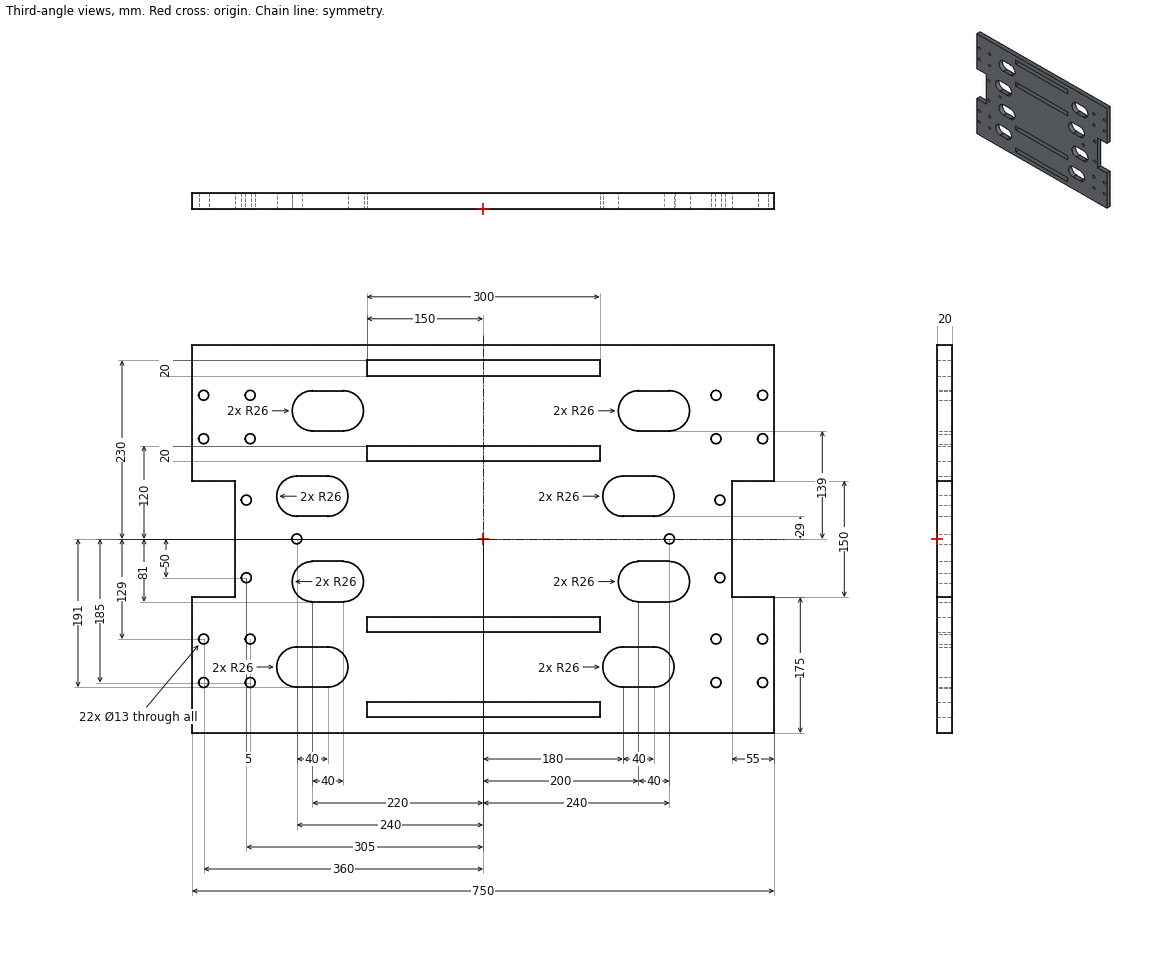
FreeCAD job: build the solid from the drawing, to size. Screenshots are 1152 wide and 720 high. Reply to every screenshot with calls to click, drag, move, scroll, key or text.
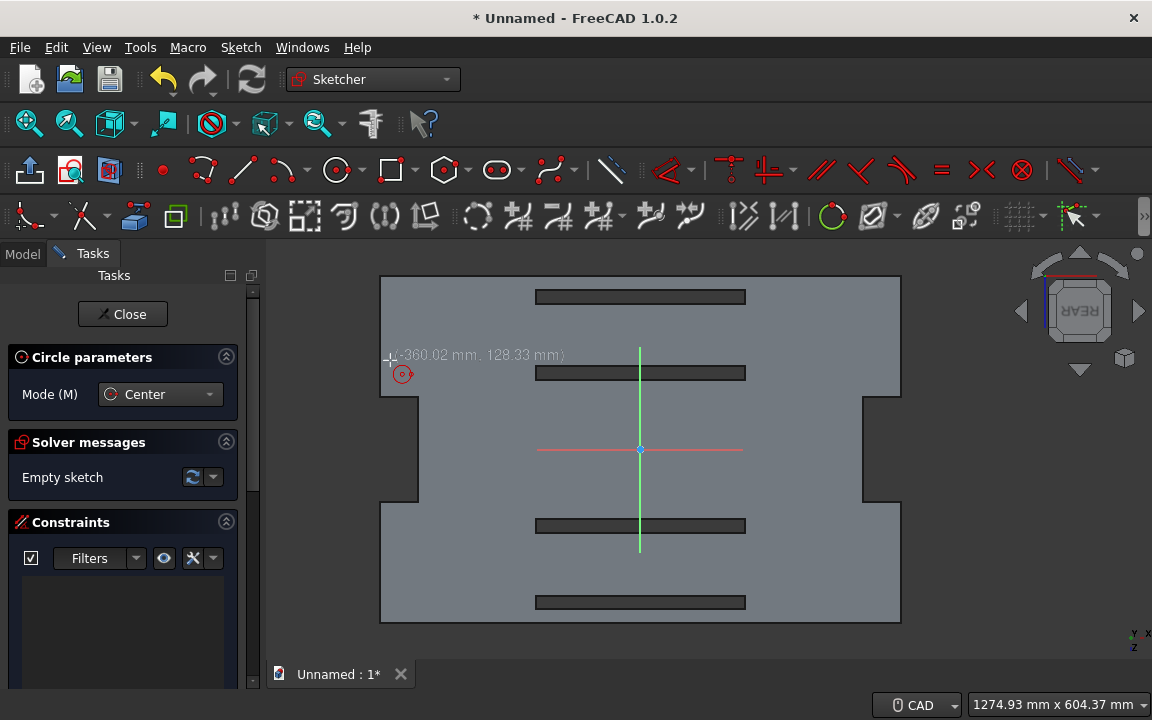
click(390, 360)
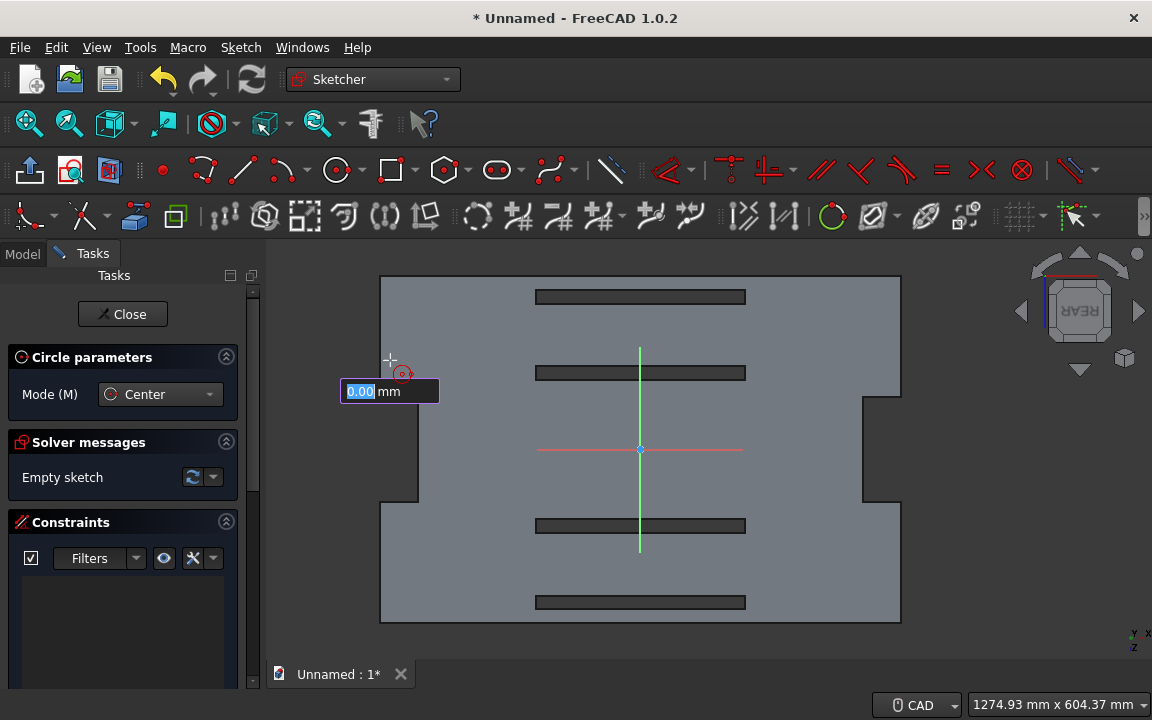
scroll(393, 357, up, 7)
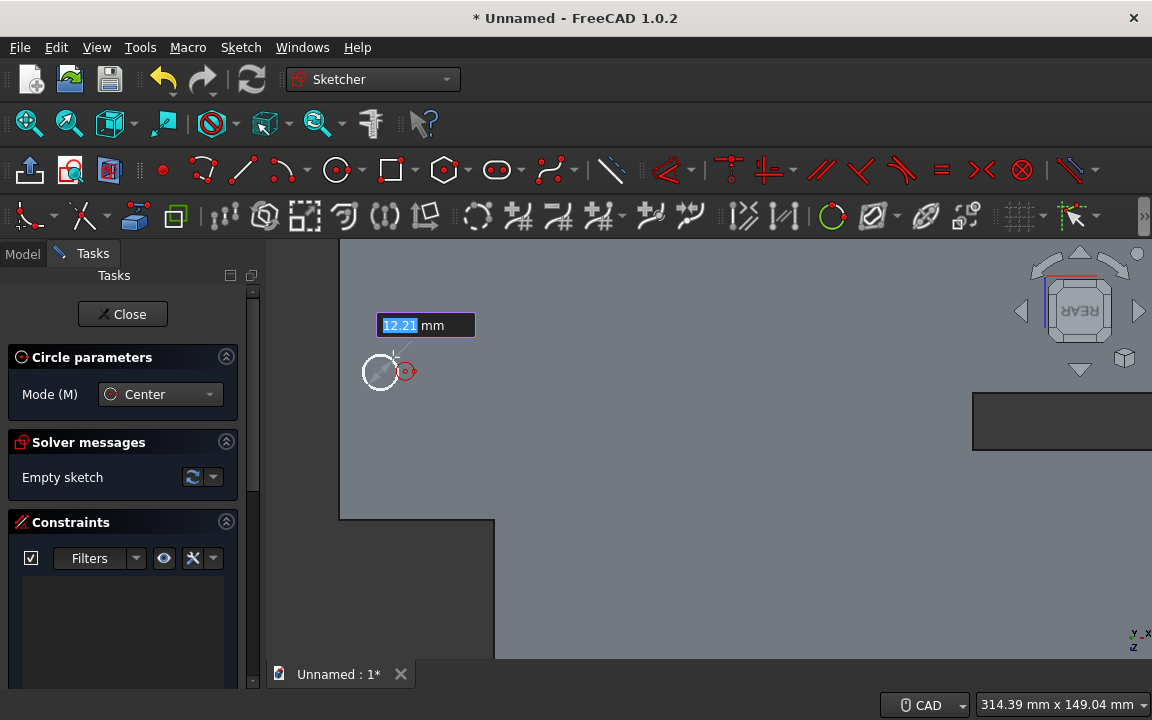
click(394, 355)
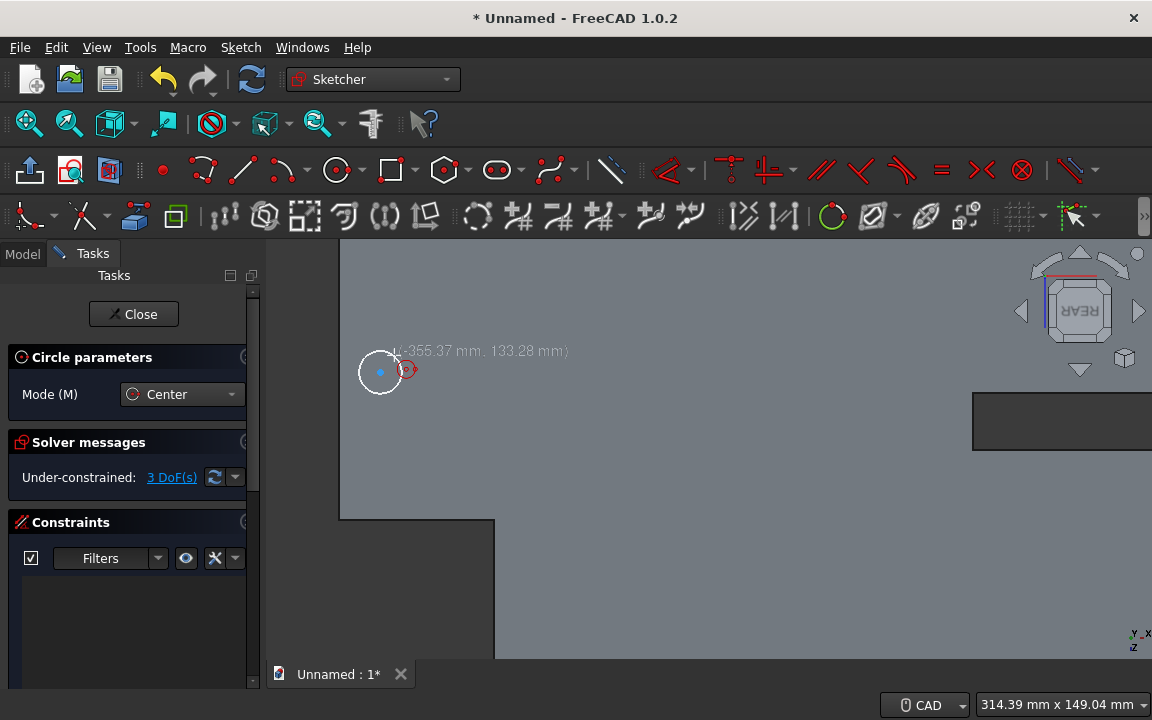
scroll(536, 591, up, 2)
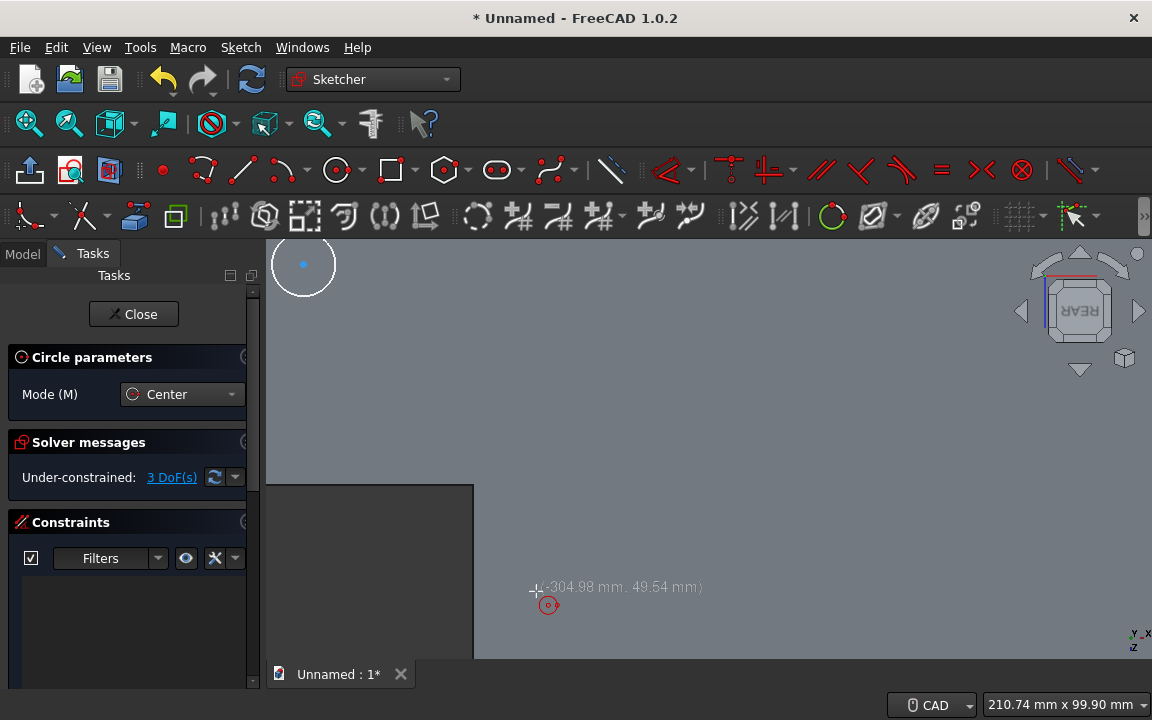
scroll(407, 379, down, 9)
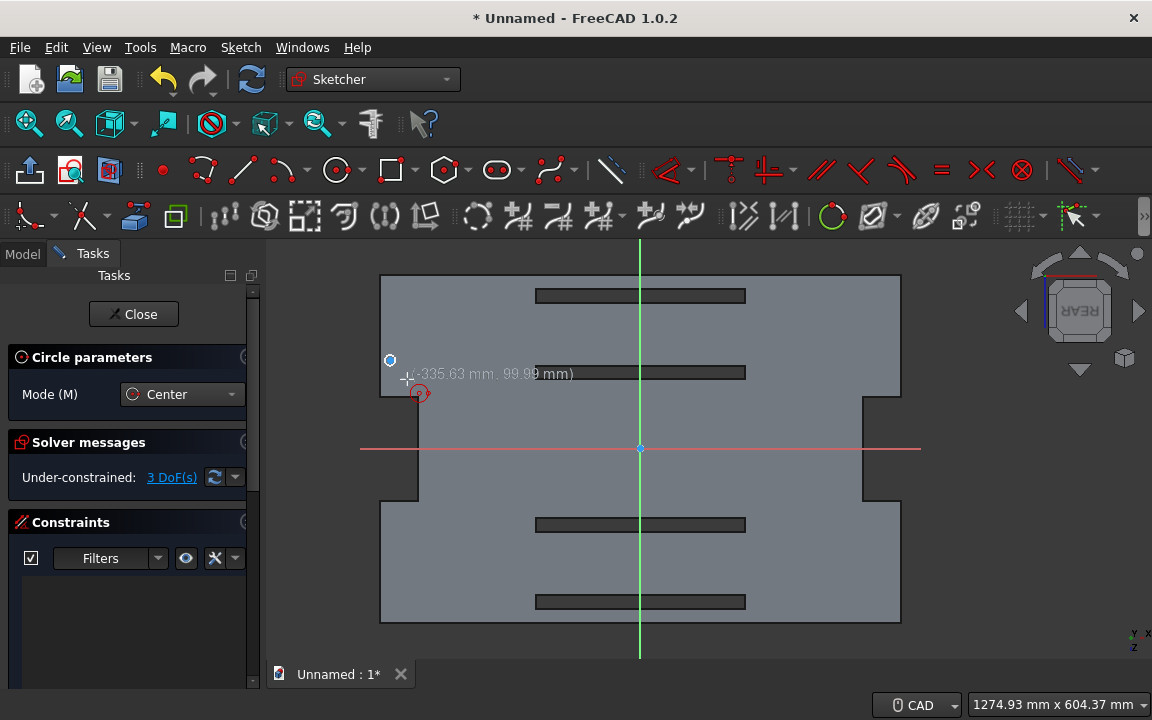
click(428, 414)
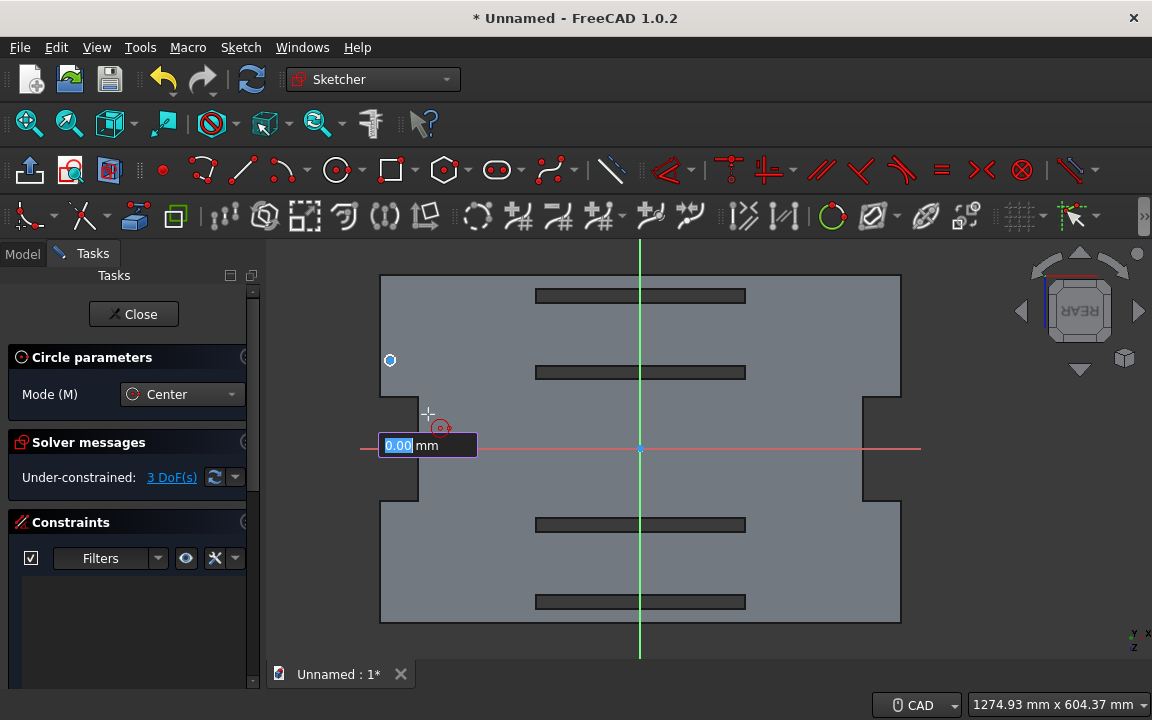
scroll(432, 411, up, 7)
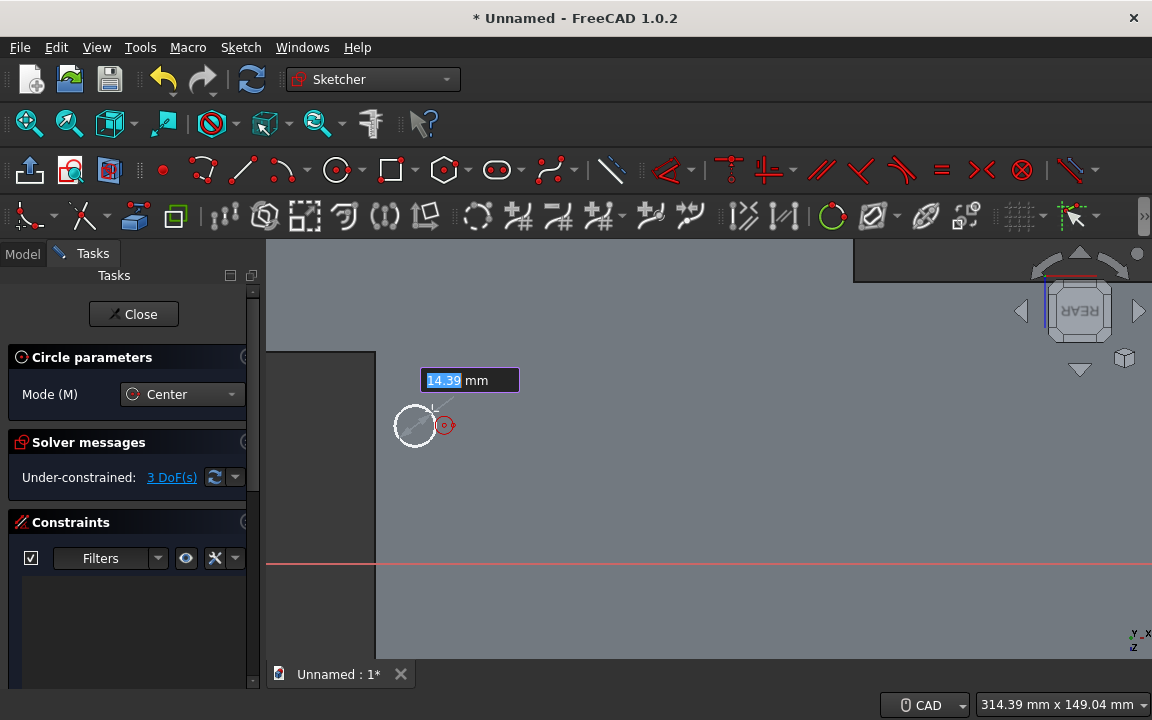
click(430, 410)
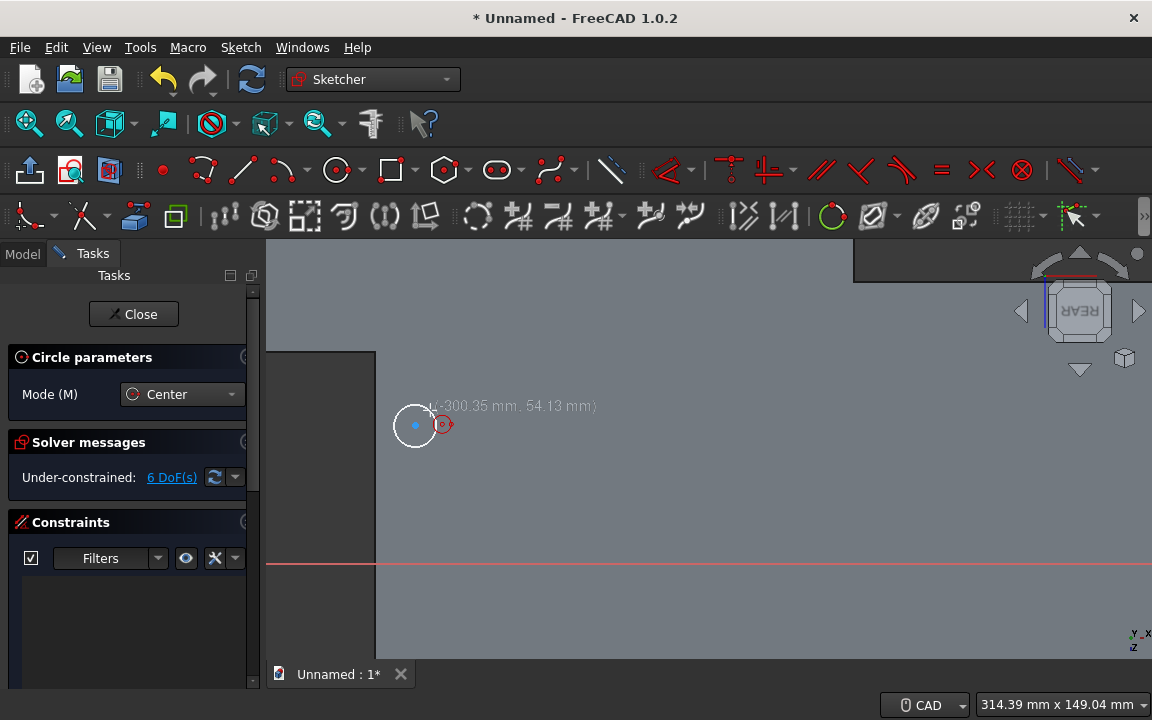
scroll(600, 564, up, 2)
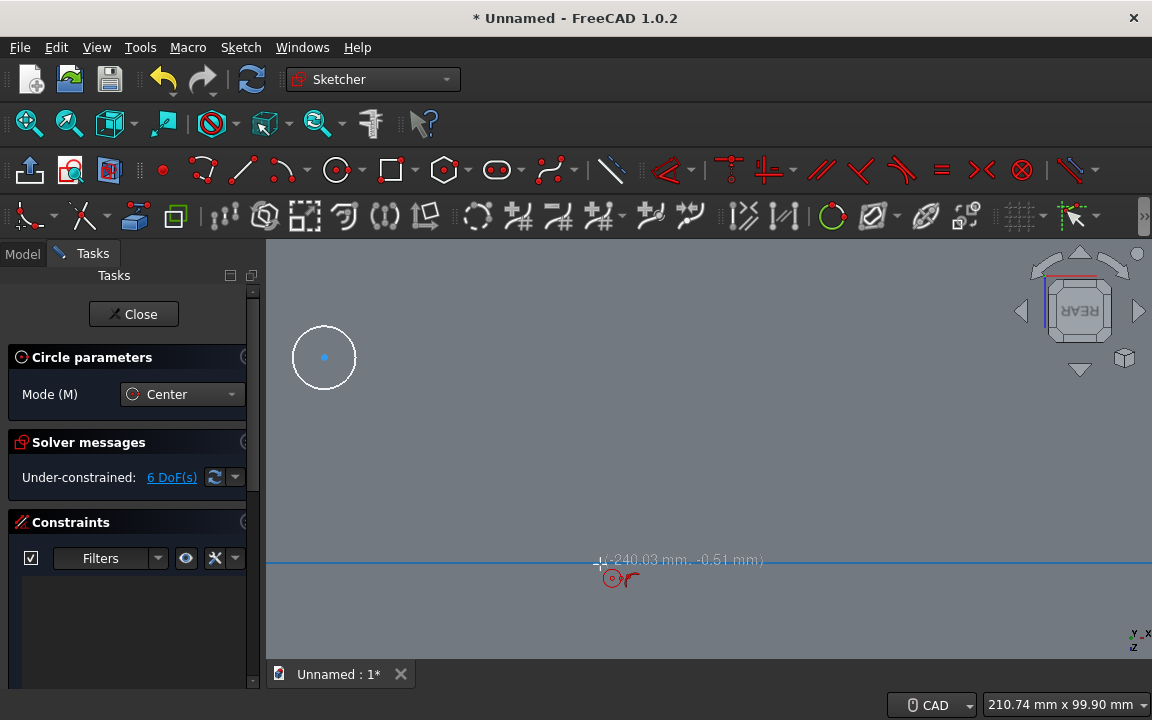
scroll(449, 426, down, 9)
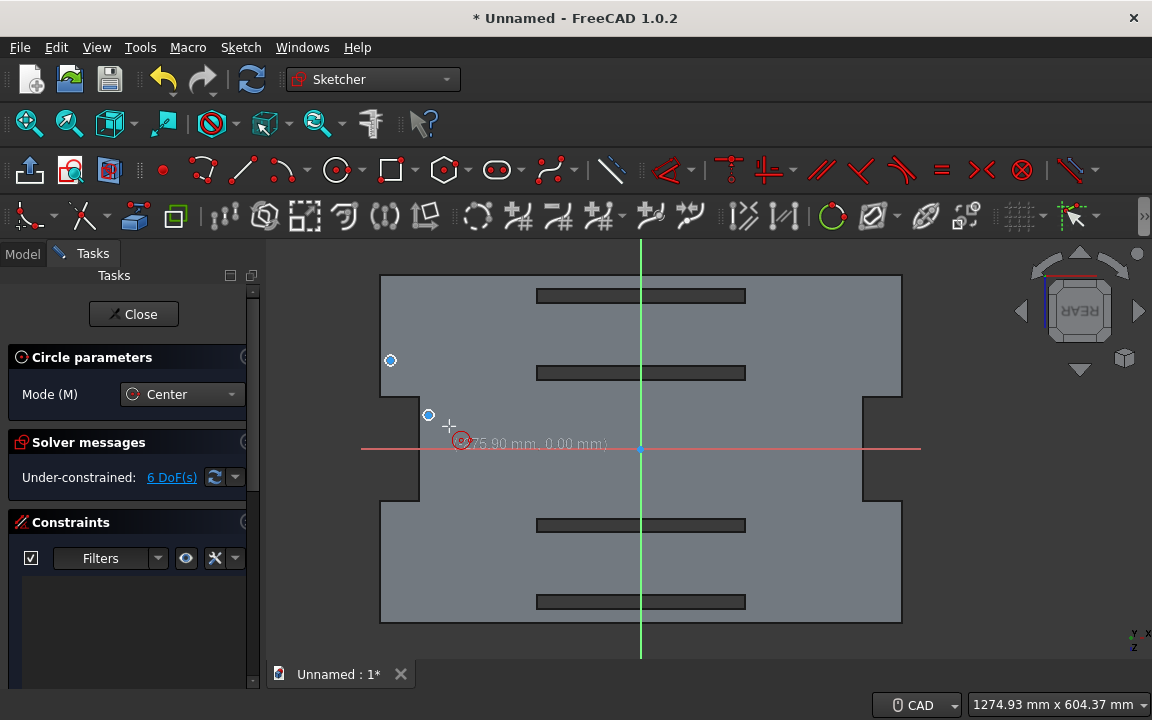
click(474, 449)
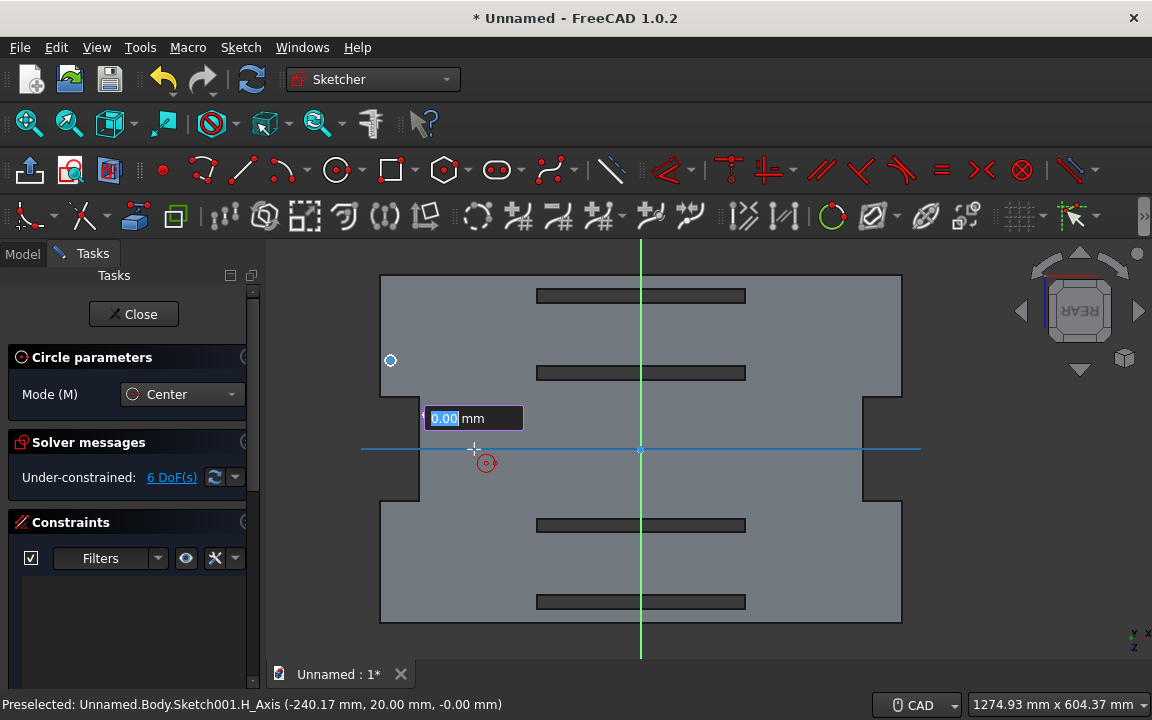
scroll(473, 453, up, 7)